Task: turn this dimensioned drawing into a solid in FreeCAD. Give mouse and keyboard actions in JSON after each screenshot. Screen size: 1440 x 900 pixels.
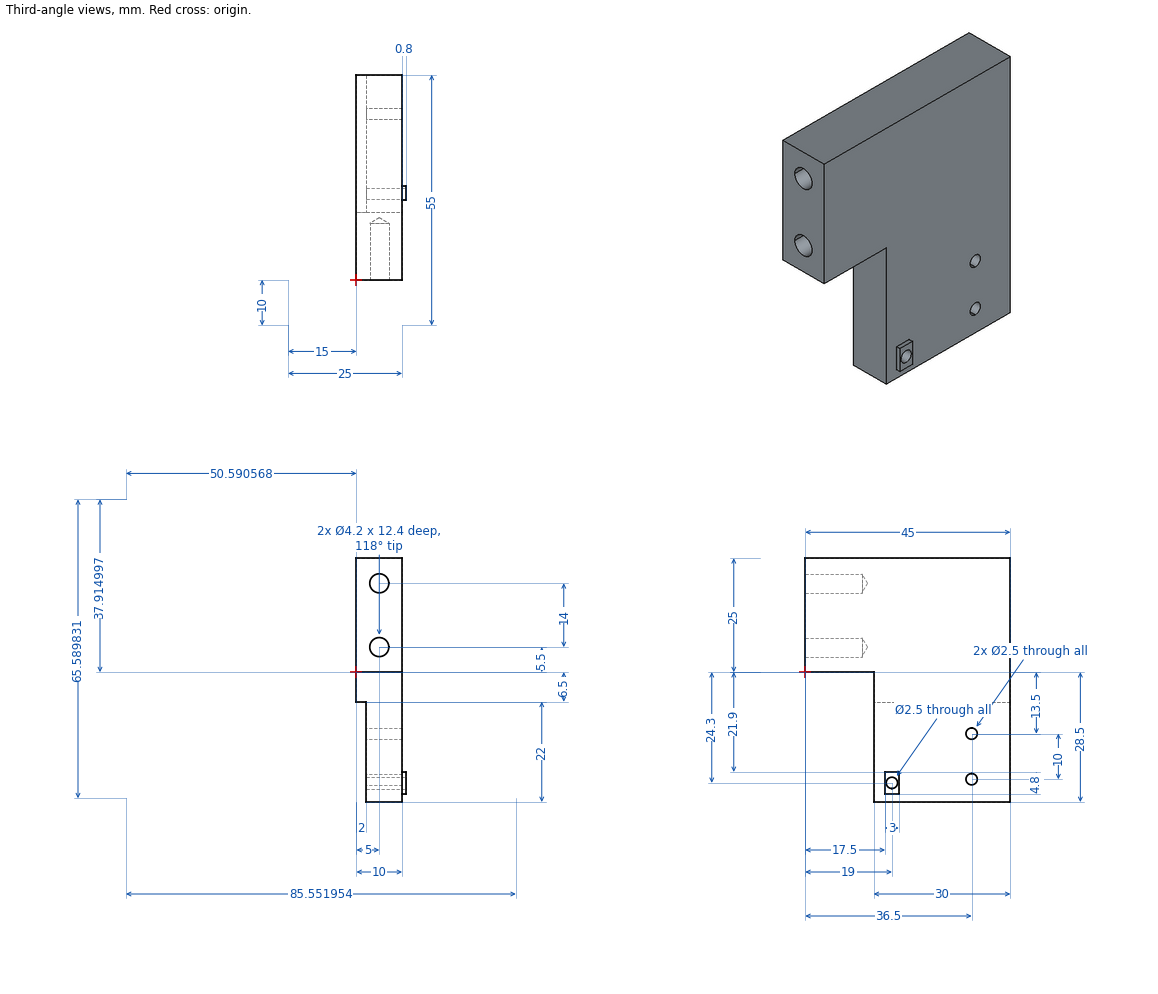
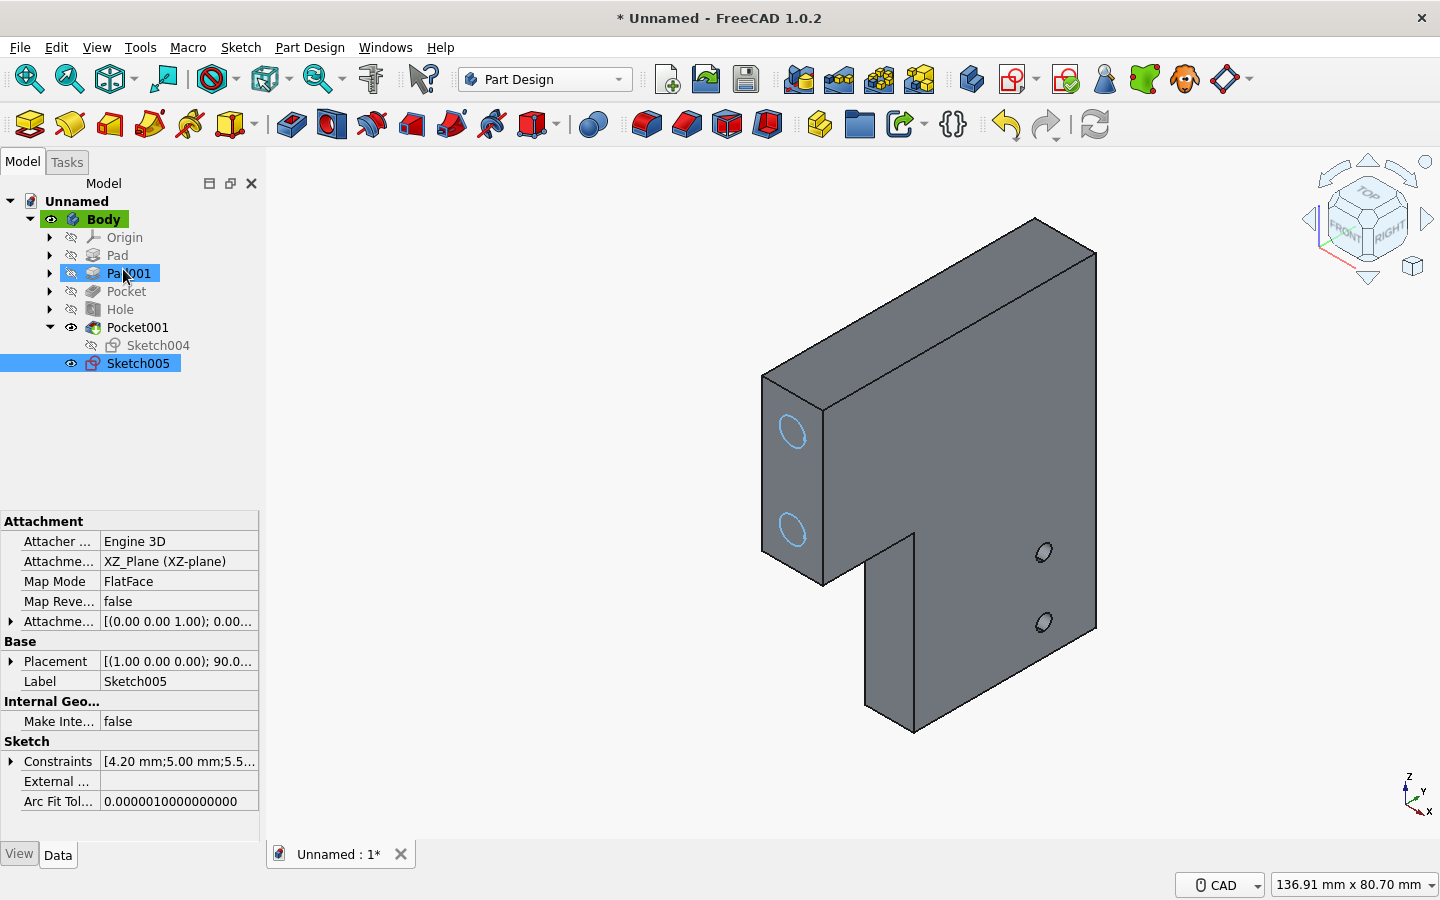
{"action": "left_click", "coordinate": [332, 124]}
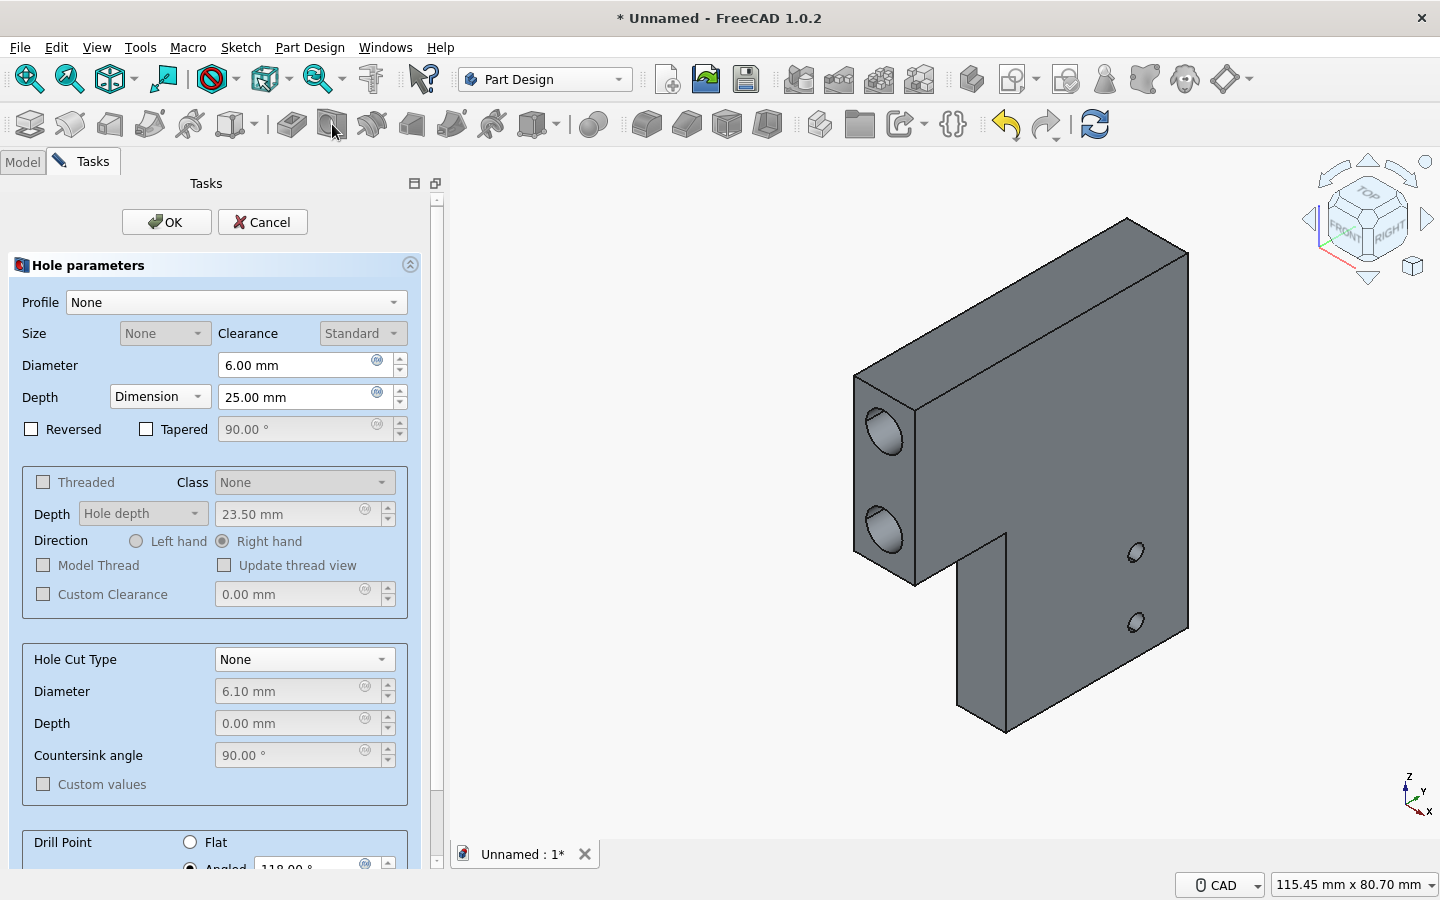
{"action": "triple_click", "coordinate": [305, 365]}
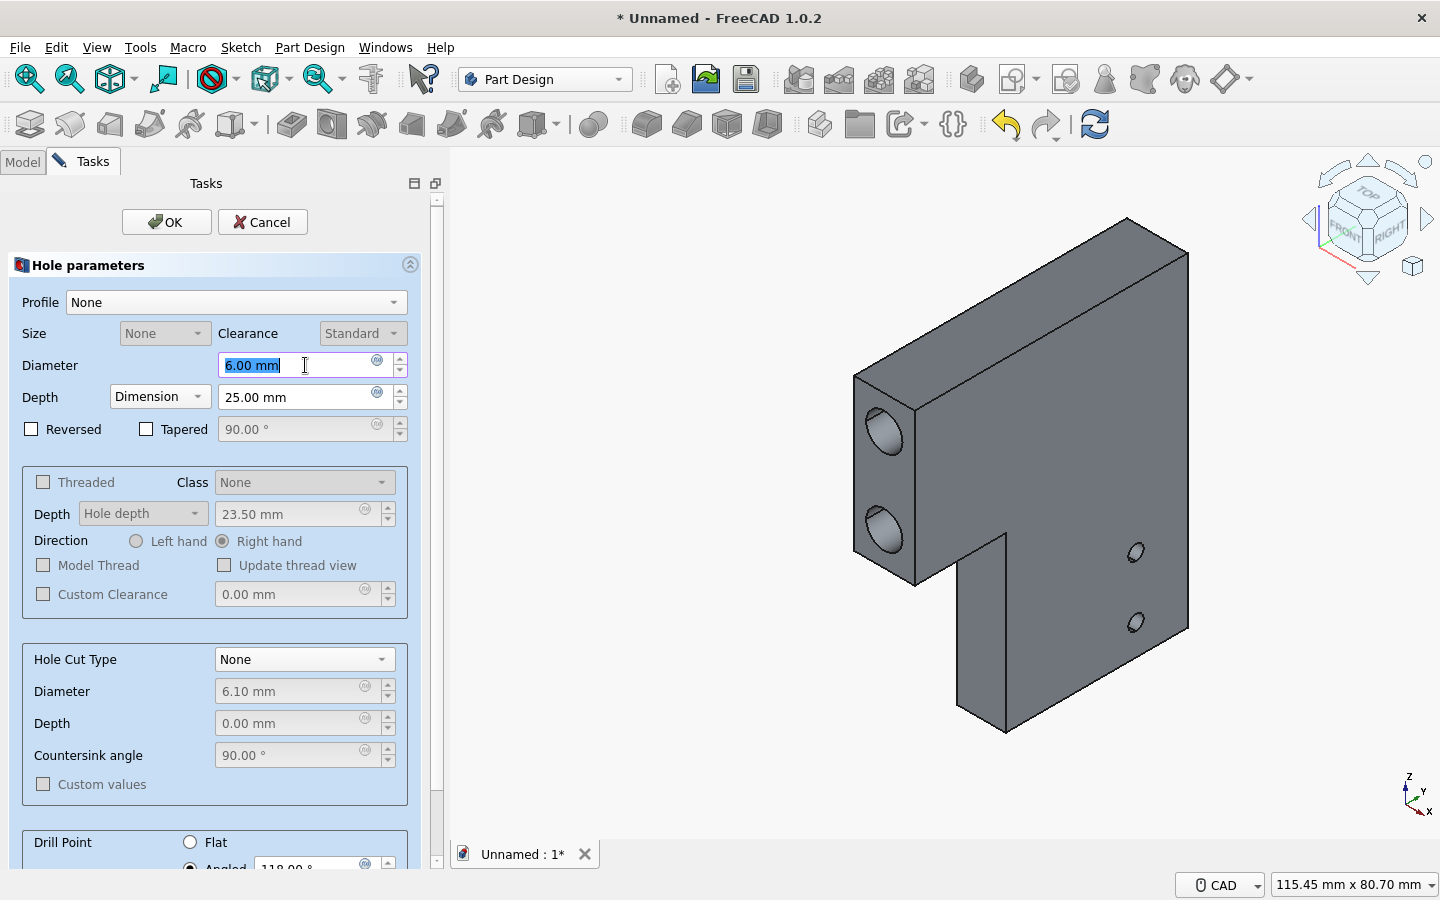
{"action": "type", "text": "4.2"}
{"action": "key", "text": "Tab"}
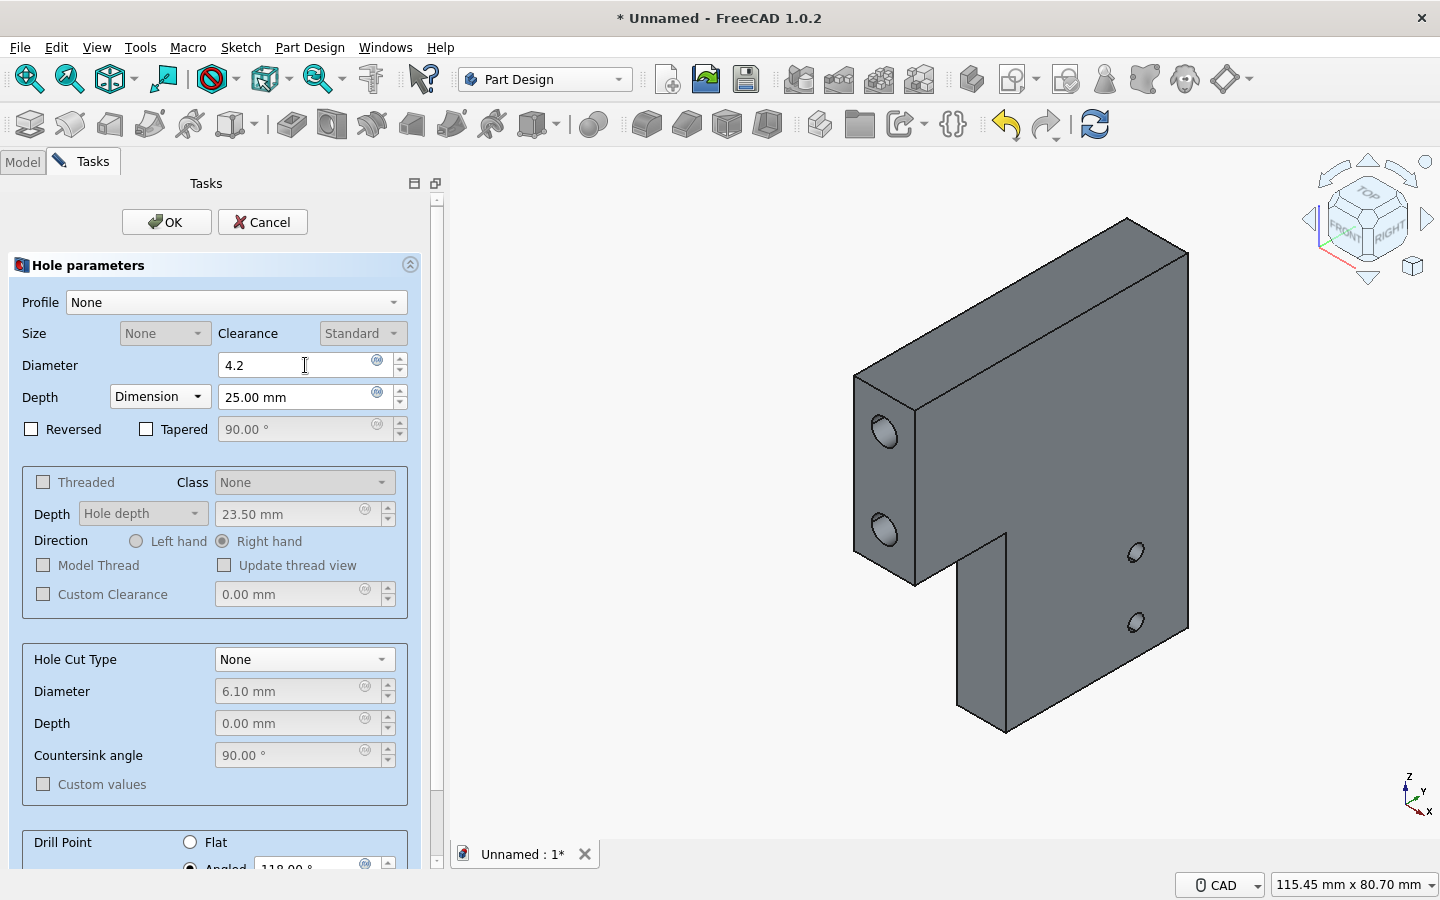
{"action": "triple_click", "coordinate": [305, 397]}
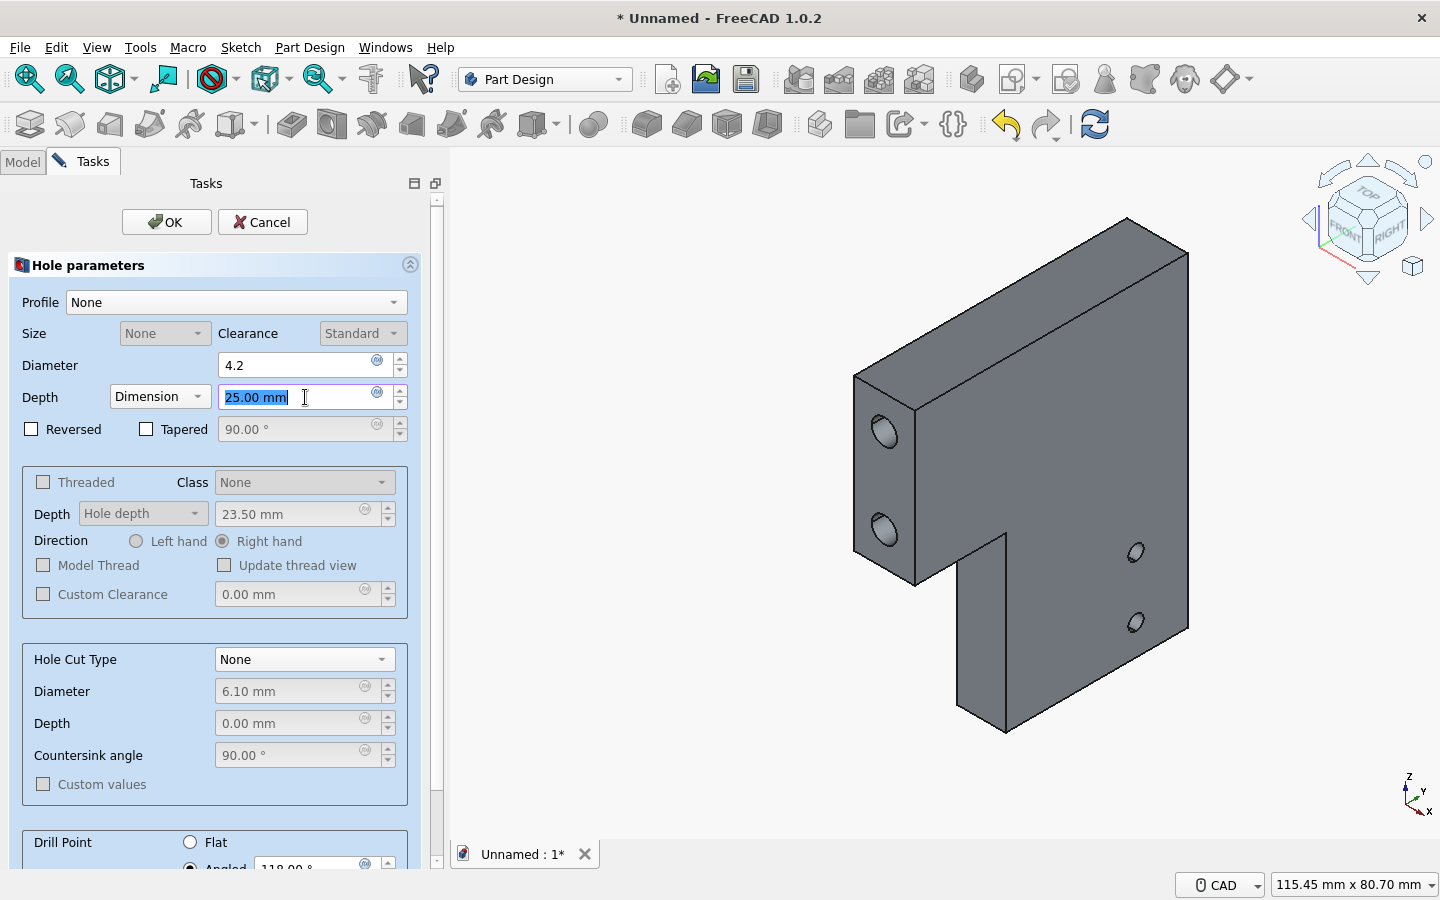
{"action": "type", "text": "12.4"}
{"action": "key", "text": "Tab"}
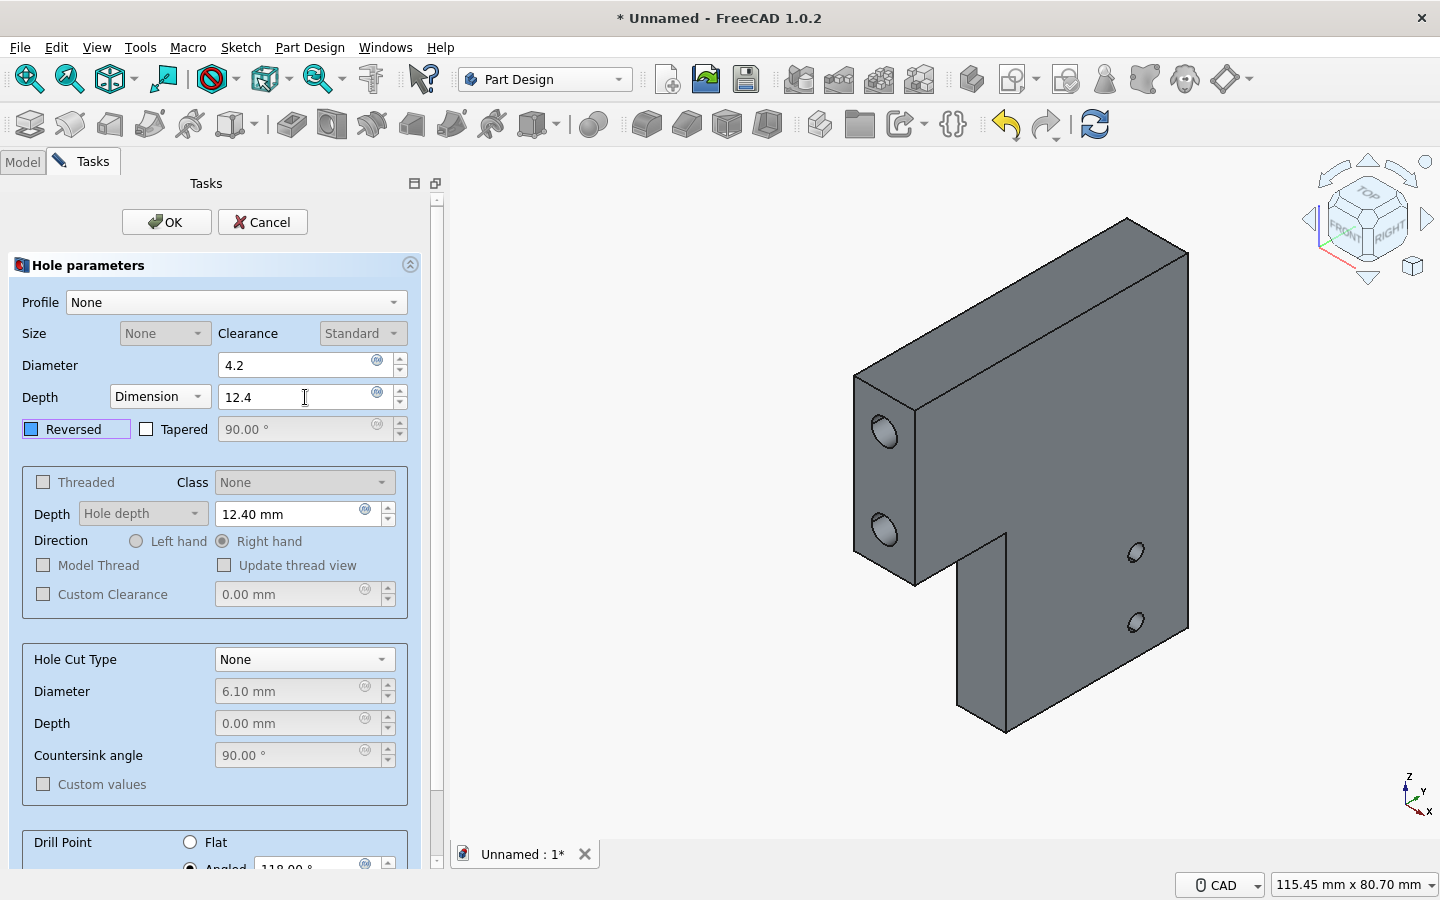
{"action": "left_click", "coordinate": [167, 222]}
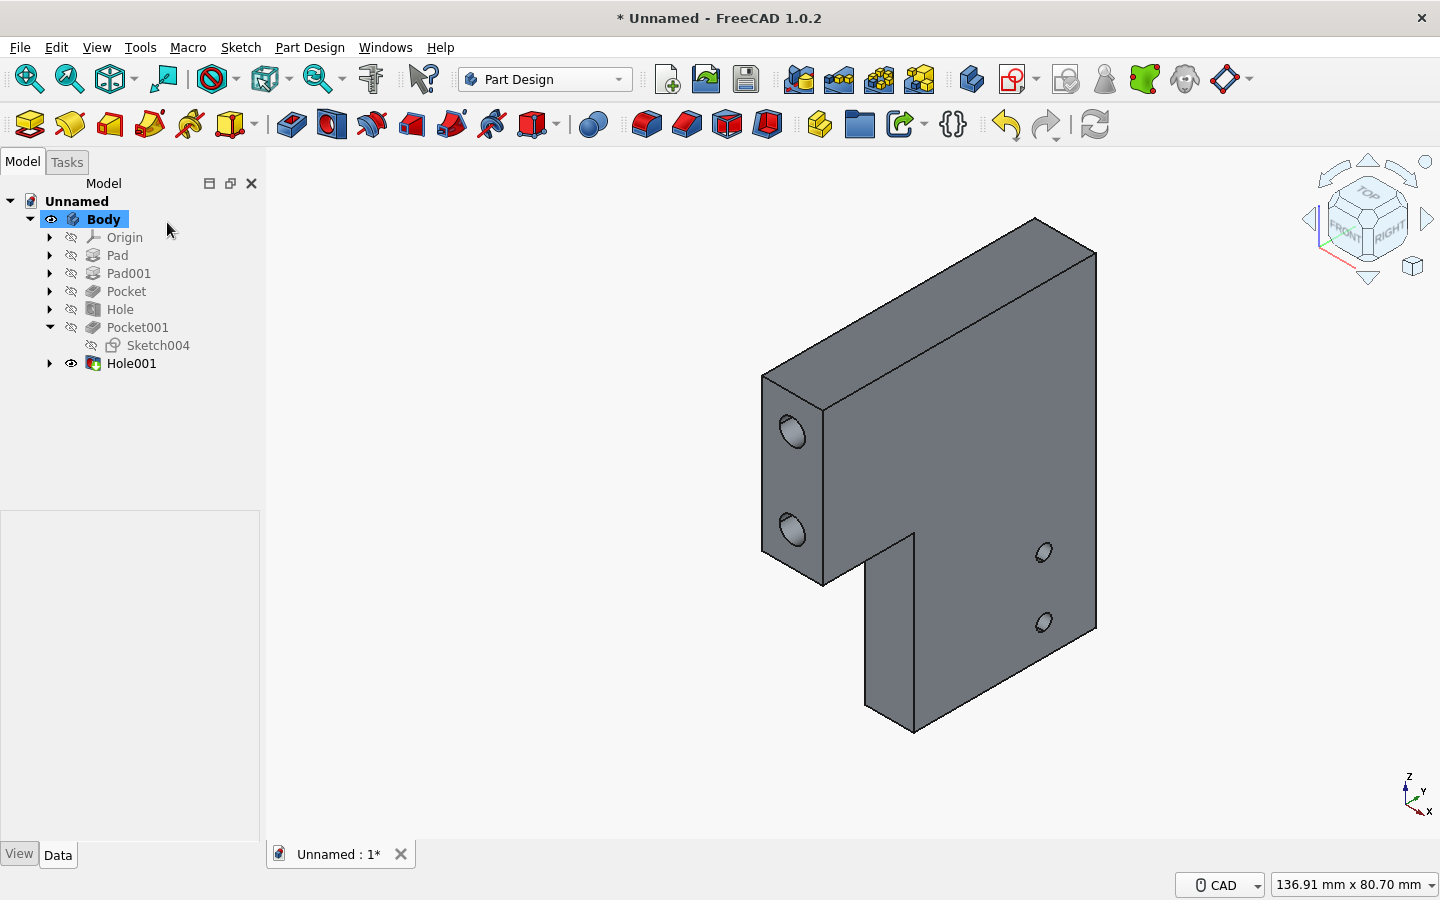
{"action": "left_click", "coordinate": [998, 442]}